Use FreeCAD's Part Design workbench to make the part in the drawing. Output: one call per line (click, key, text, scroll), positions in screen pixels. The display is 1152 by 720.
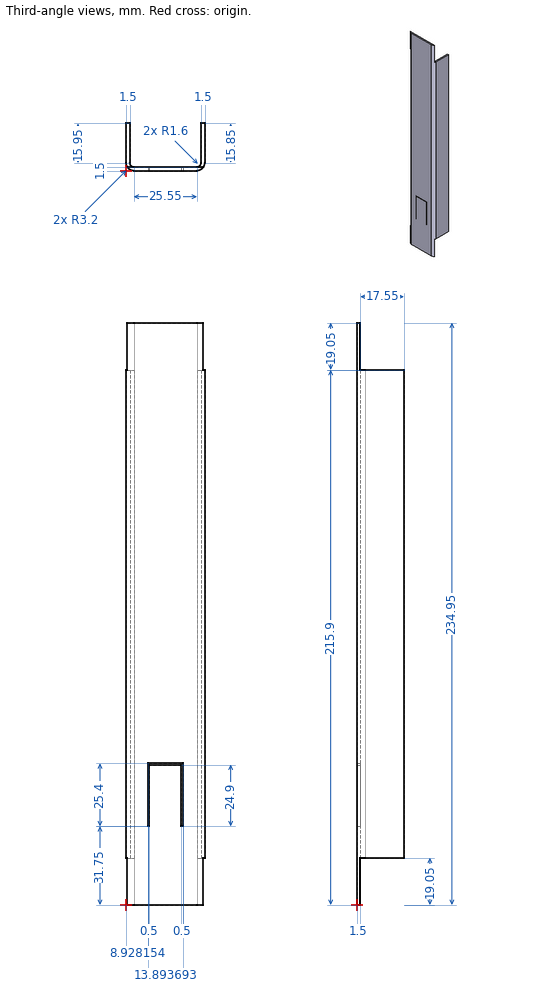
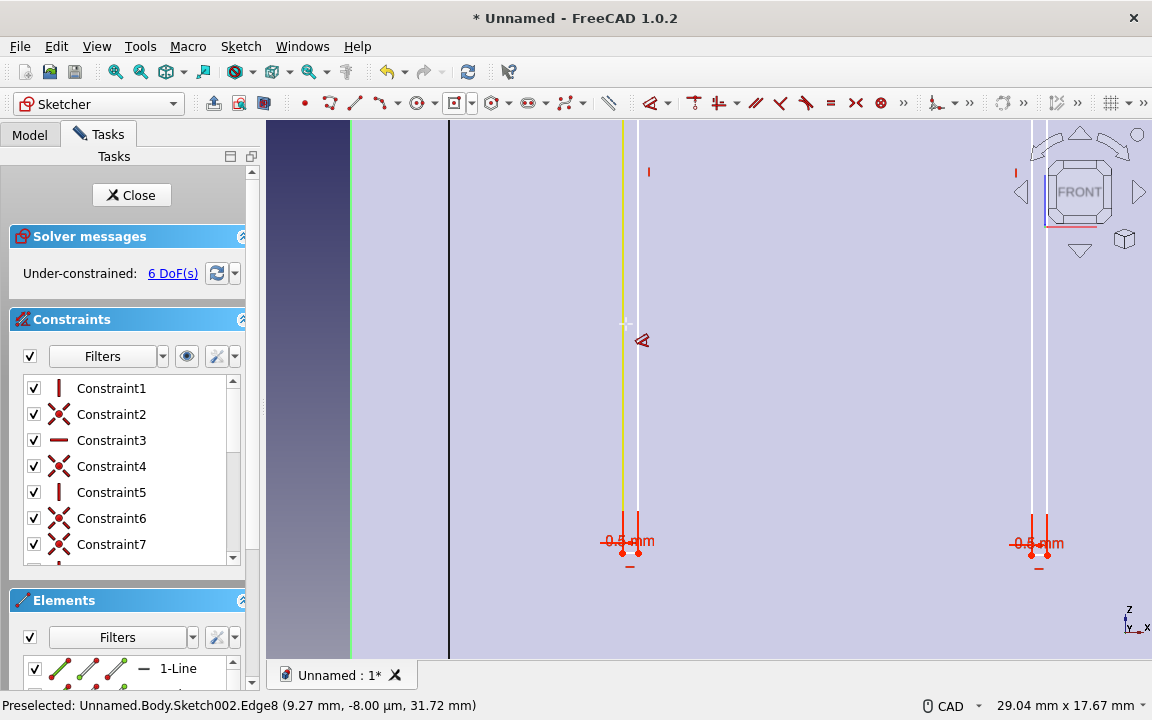
click(623, 322)
click(589, 351)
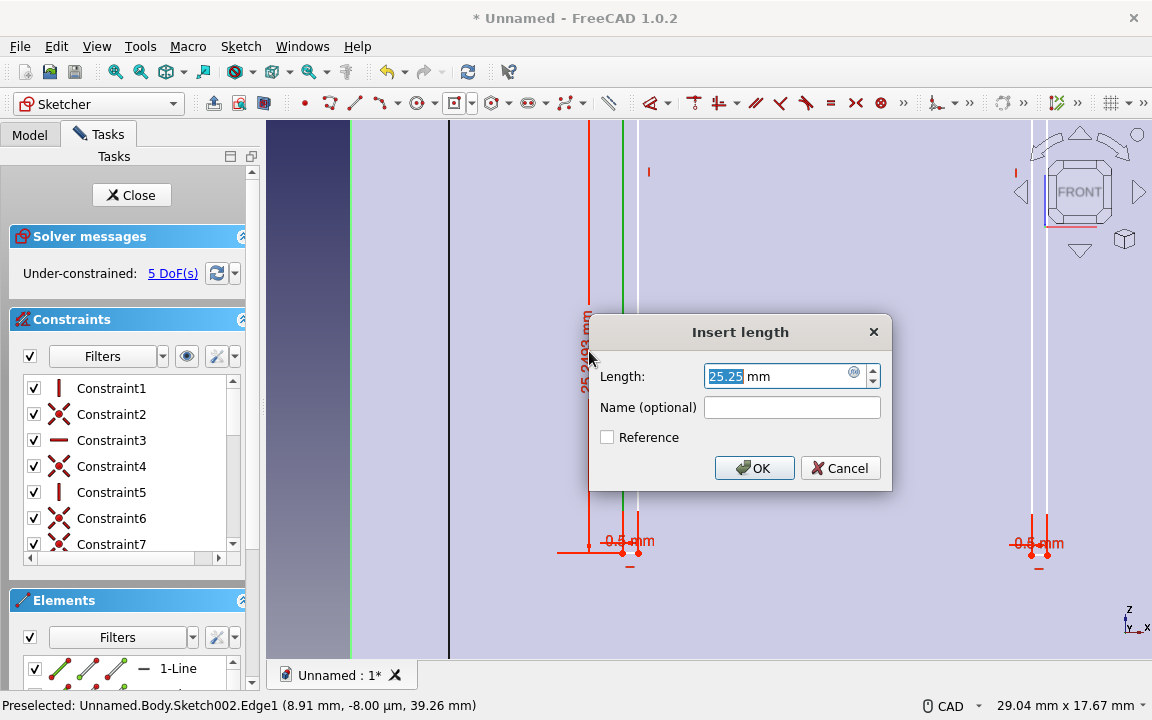
text(25.4)
key(Return)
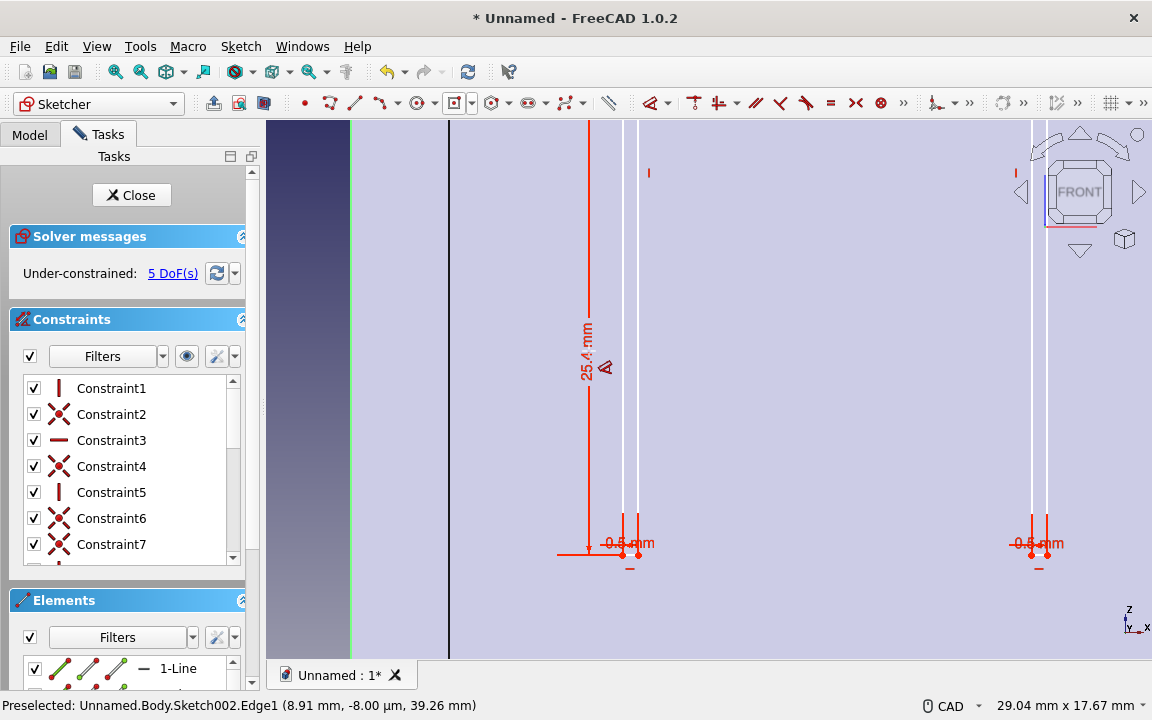
scroll(626, 324, down, 8)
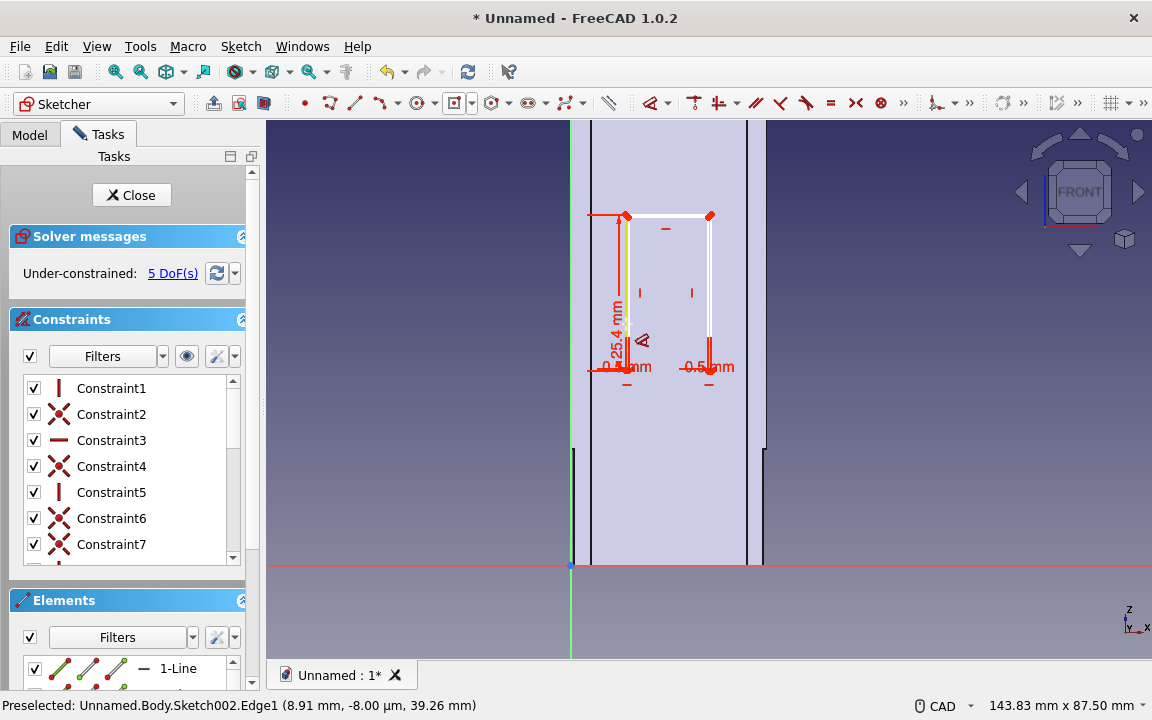
scroll(711, 261, up, 8)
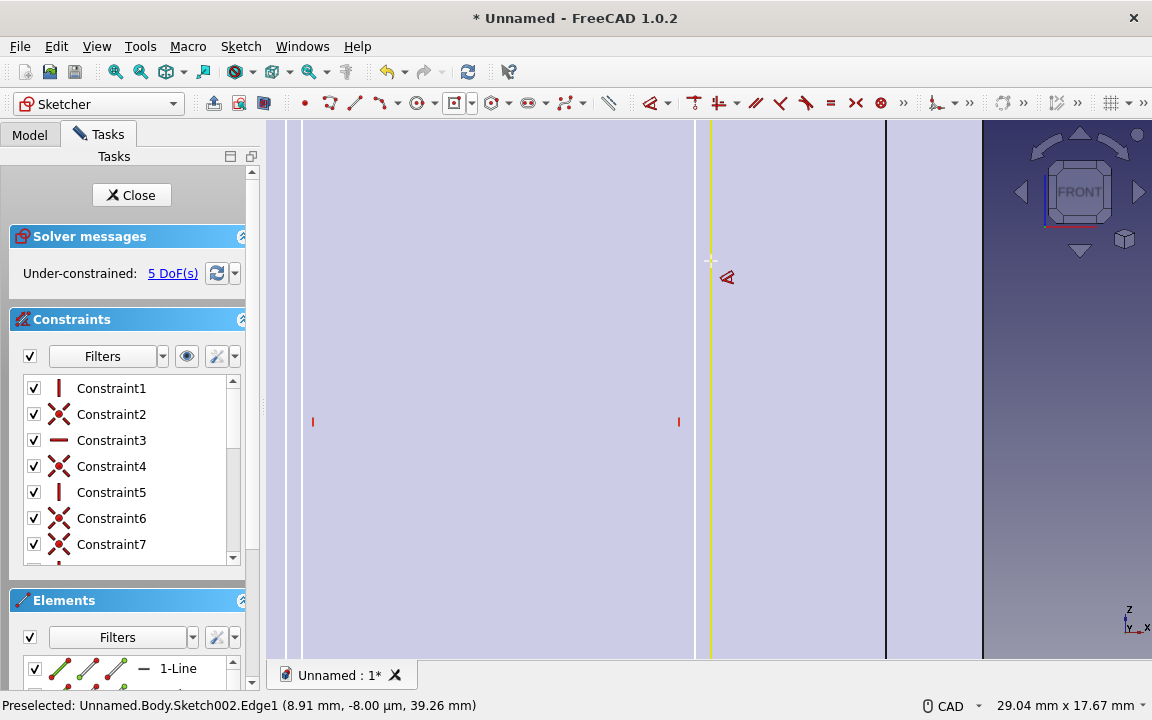
click(711, 262)
click(745, 390)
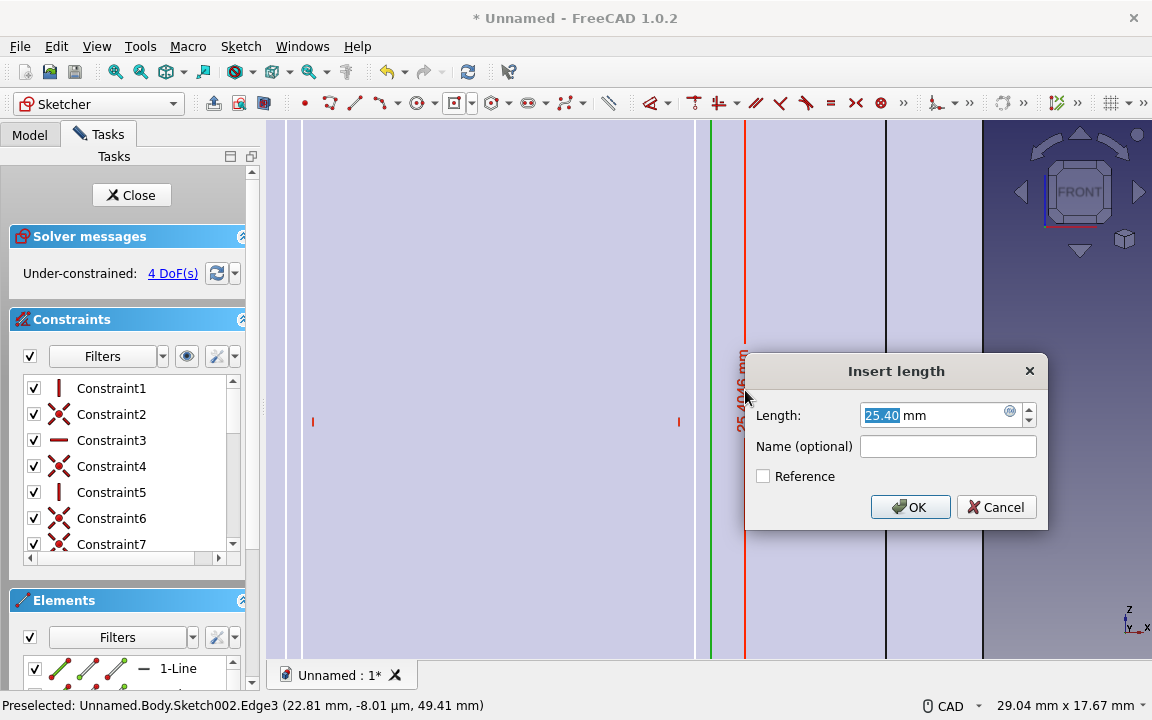
text(25.4)
key(Return)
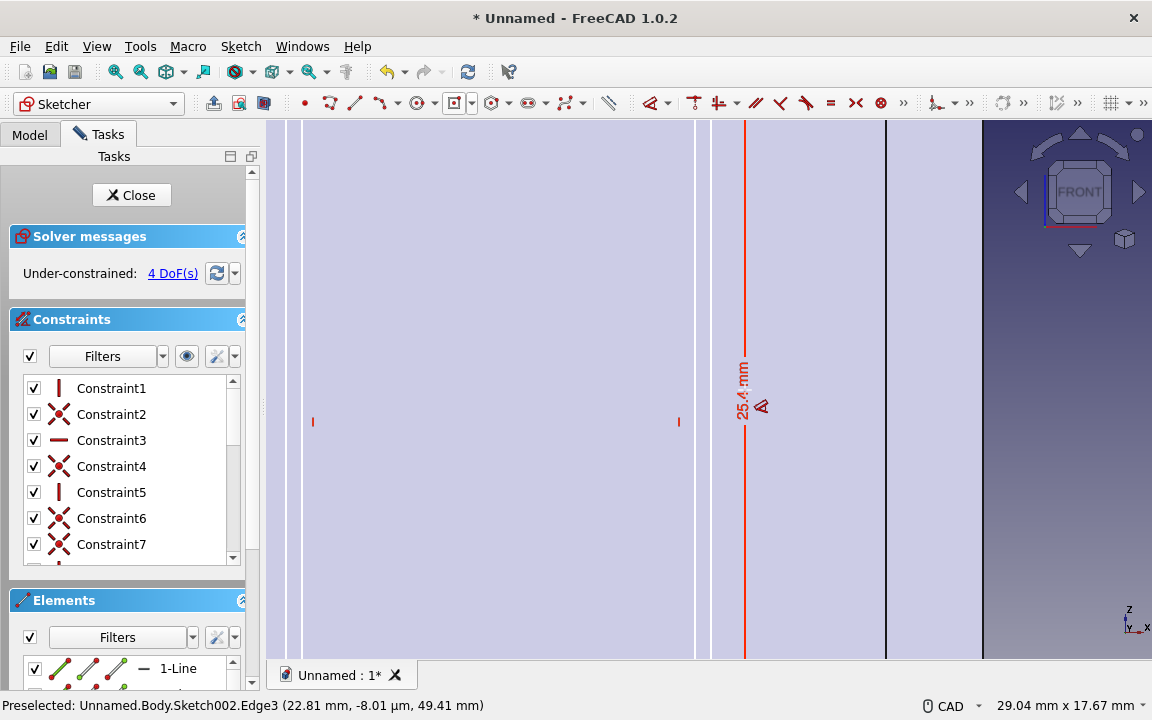
click(695, 576)
click(729, 278)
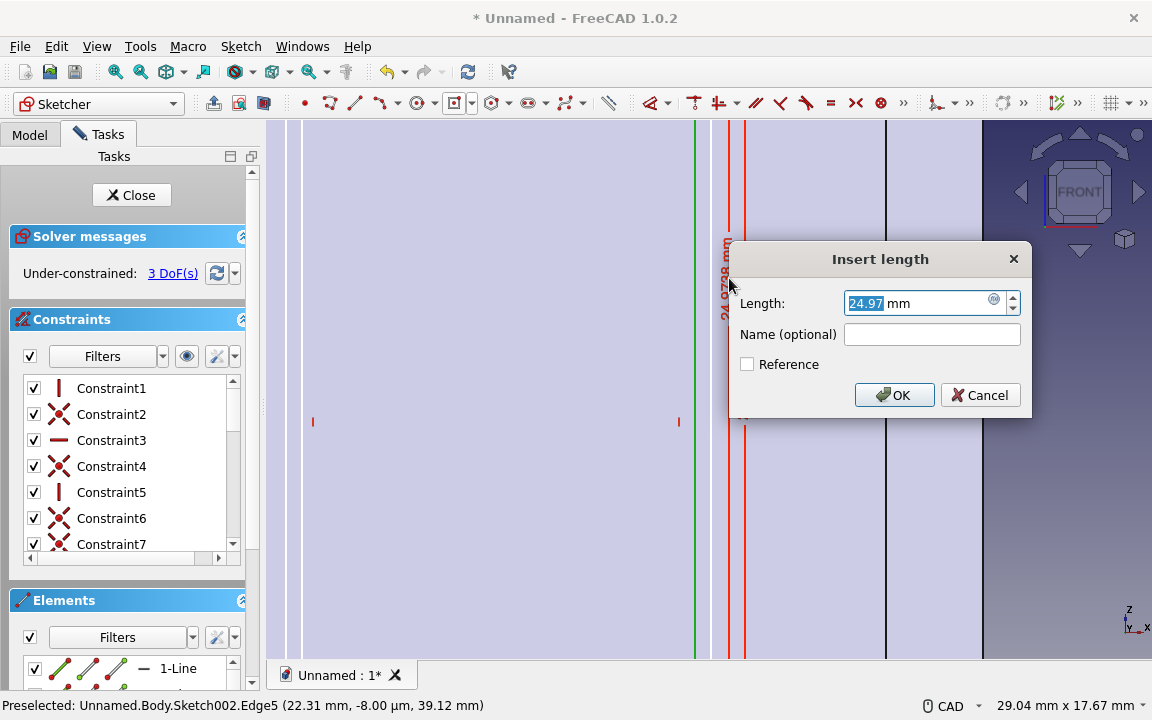
text(24.9)
key(Return)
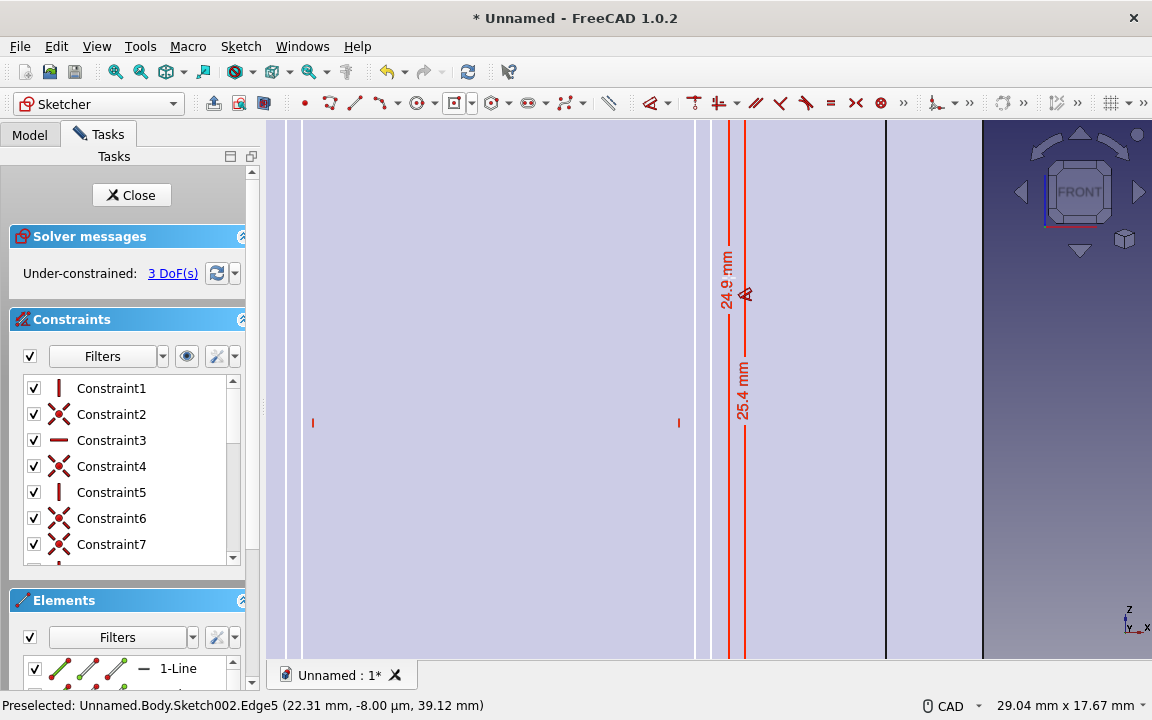
scroll(711, 261, down, 8)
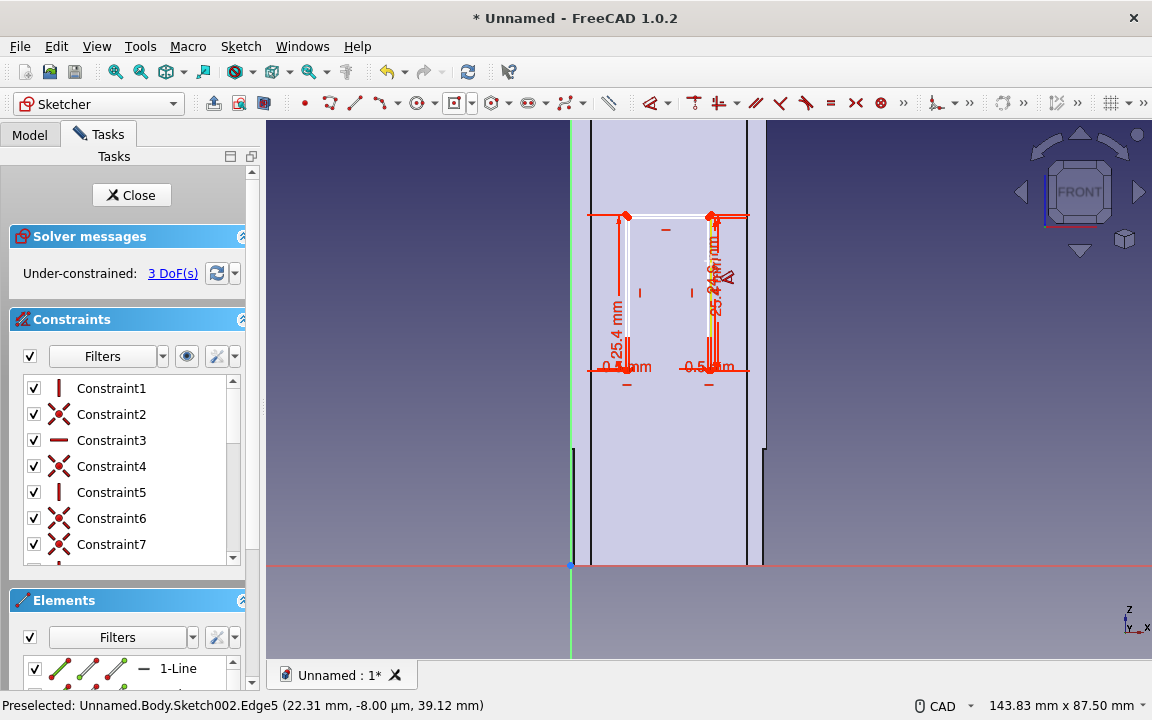
scroll(626, 371, up, 7)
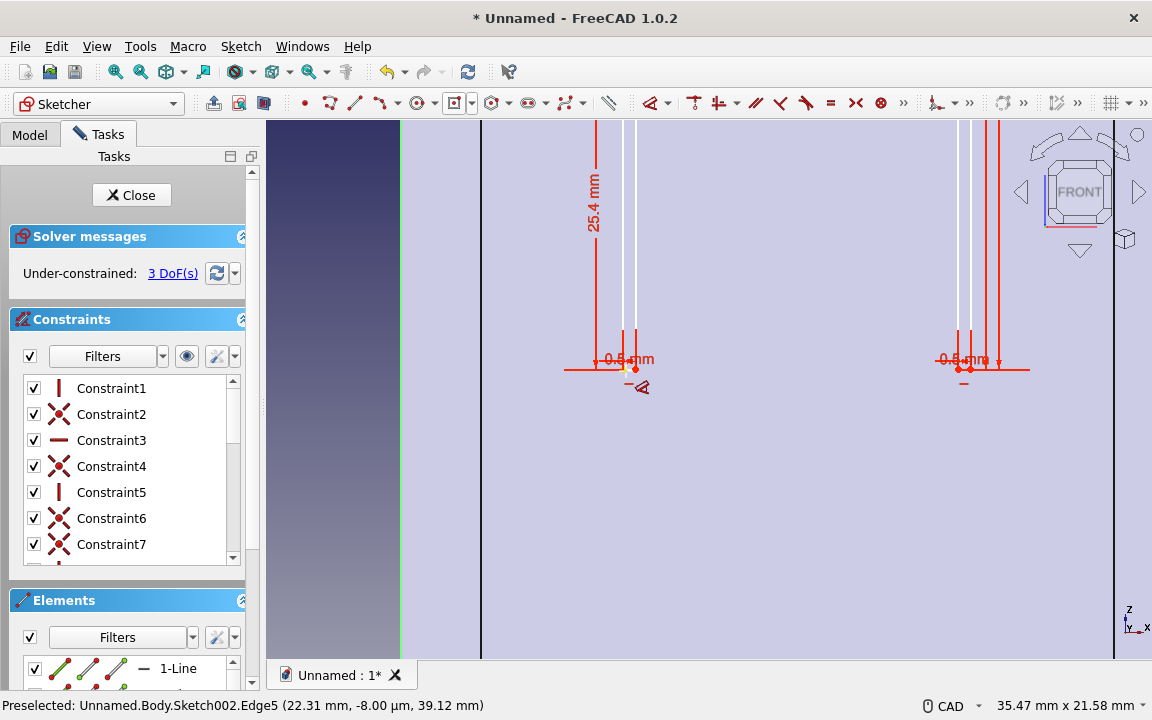
click(623, 370)
click(367, 500)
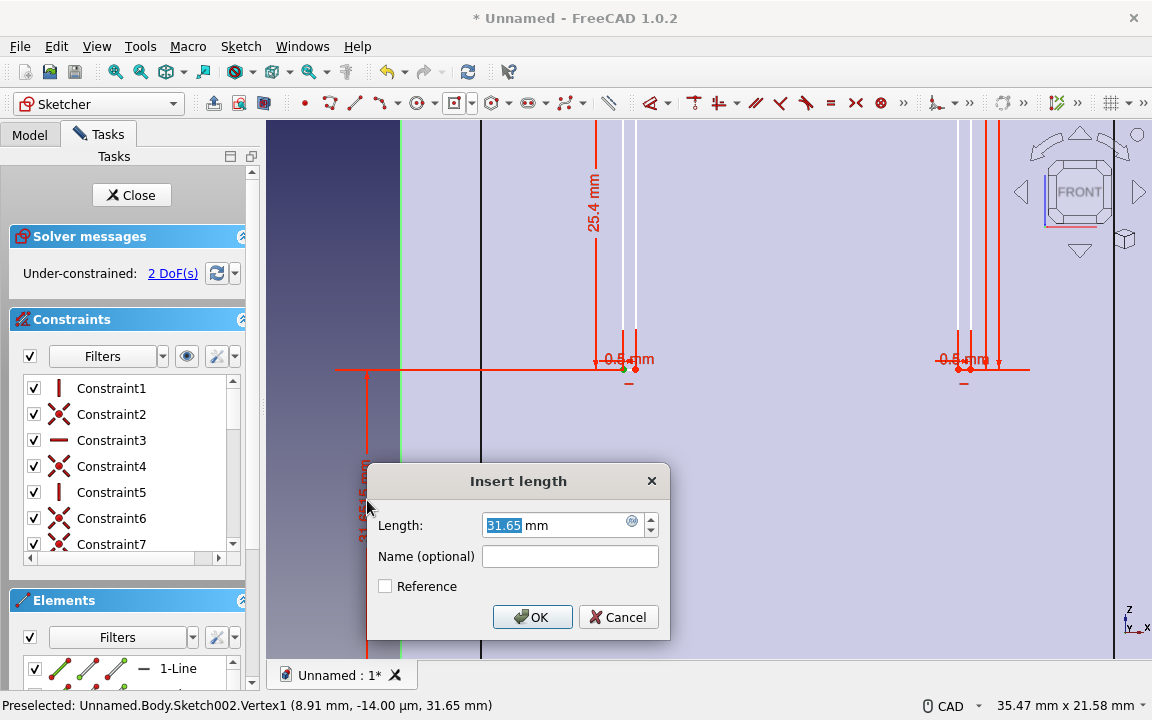
text(31.75)
key(Return)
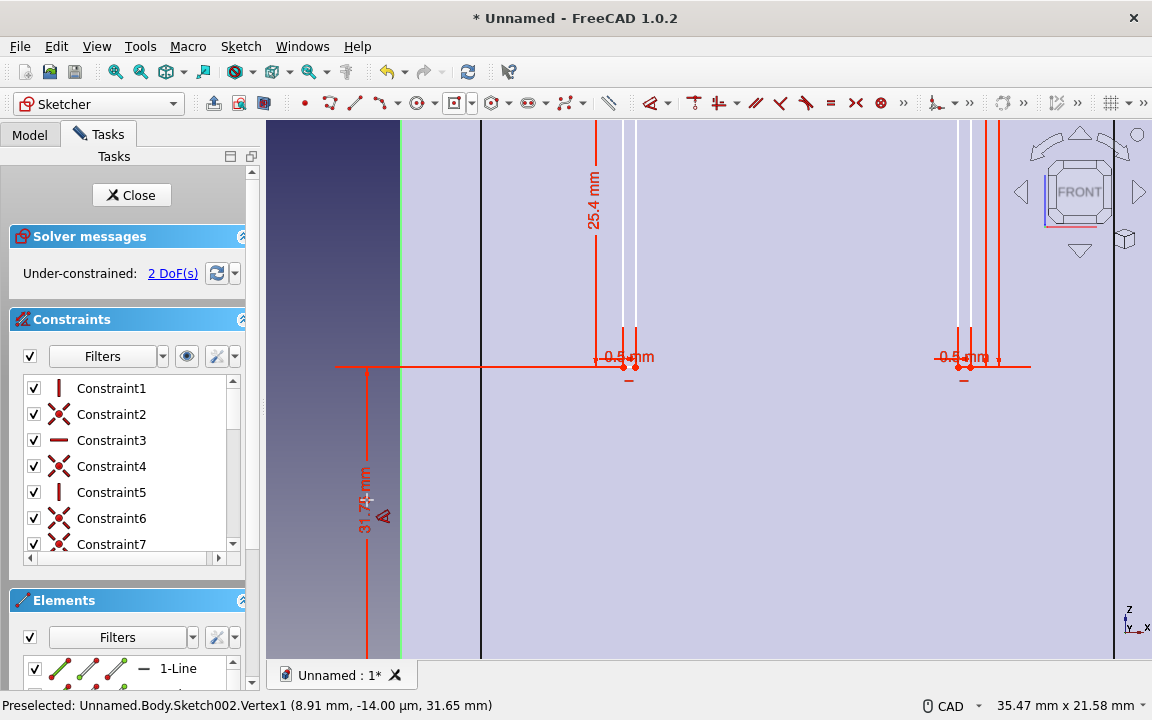
scroll(626, 371, down, 7)